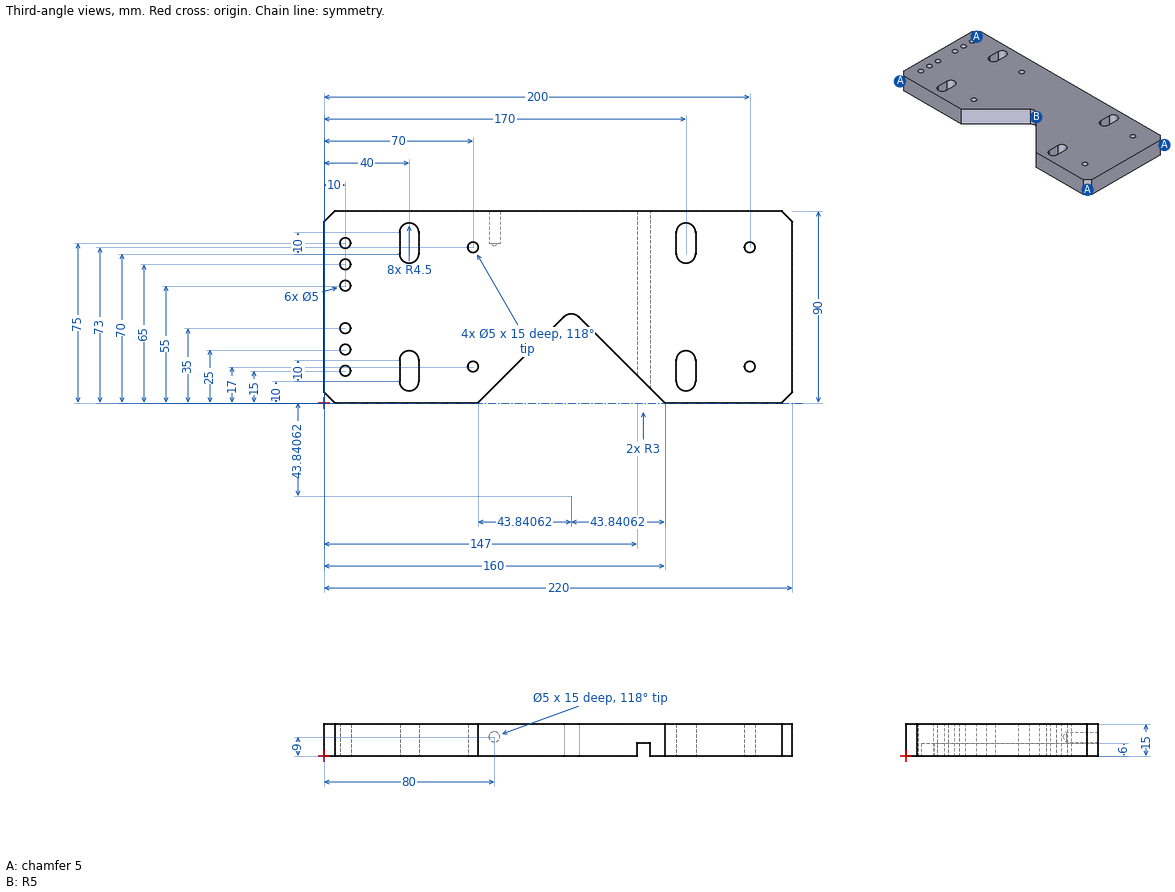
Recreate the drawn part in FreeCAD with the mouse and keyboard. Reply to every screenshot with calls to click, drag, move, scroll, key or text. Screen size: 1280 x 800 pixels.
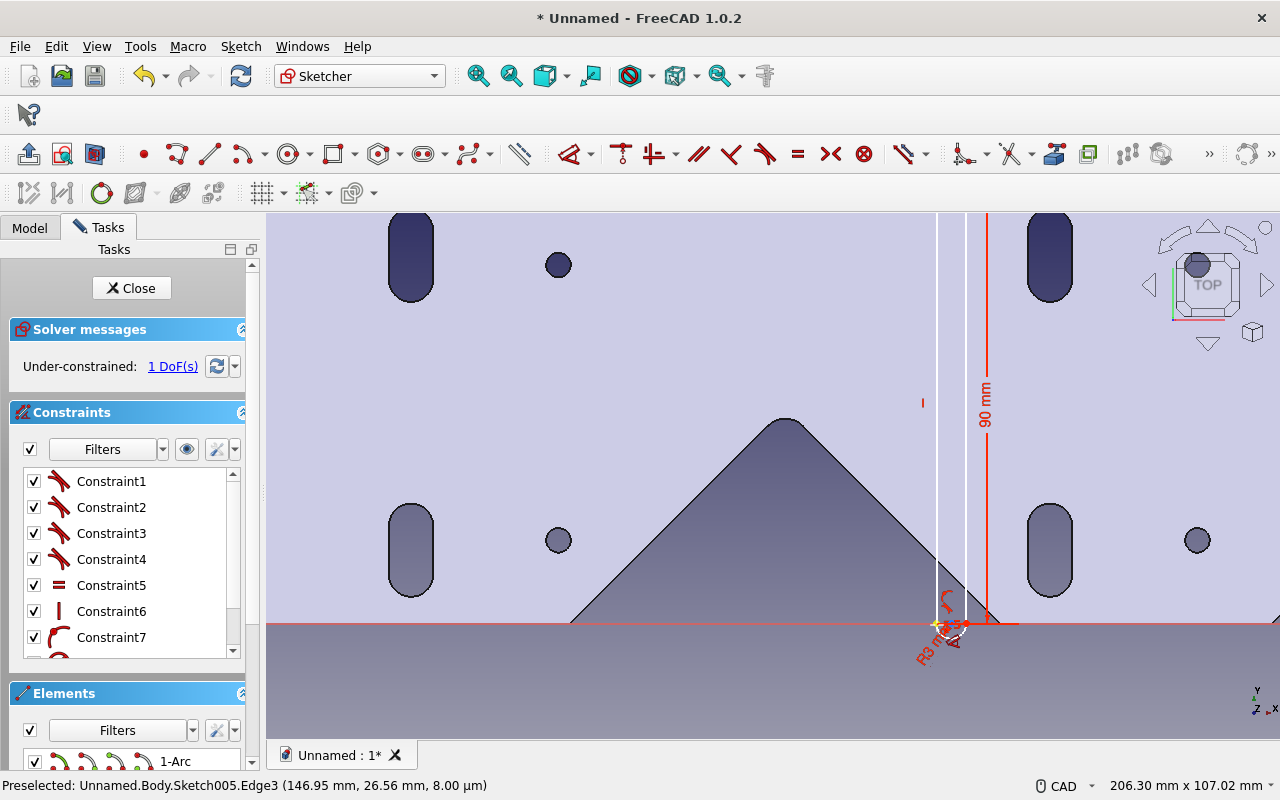
click(937, 624)
click(615, 658)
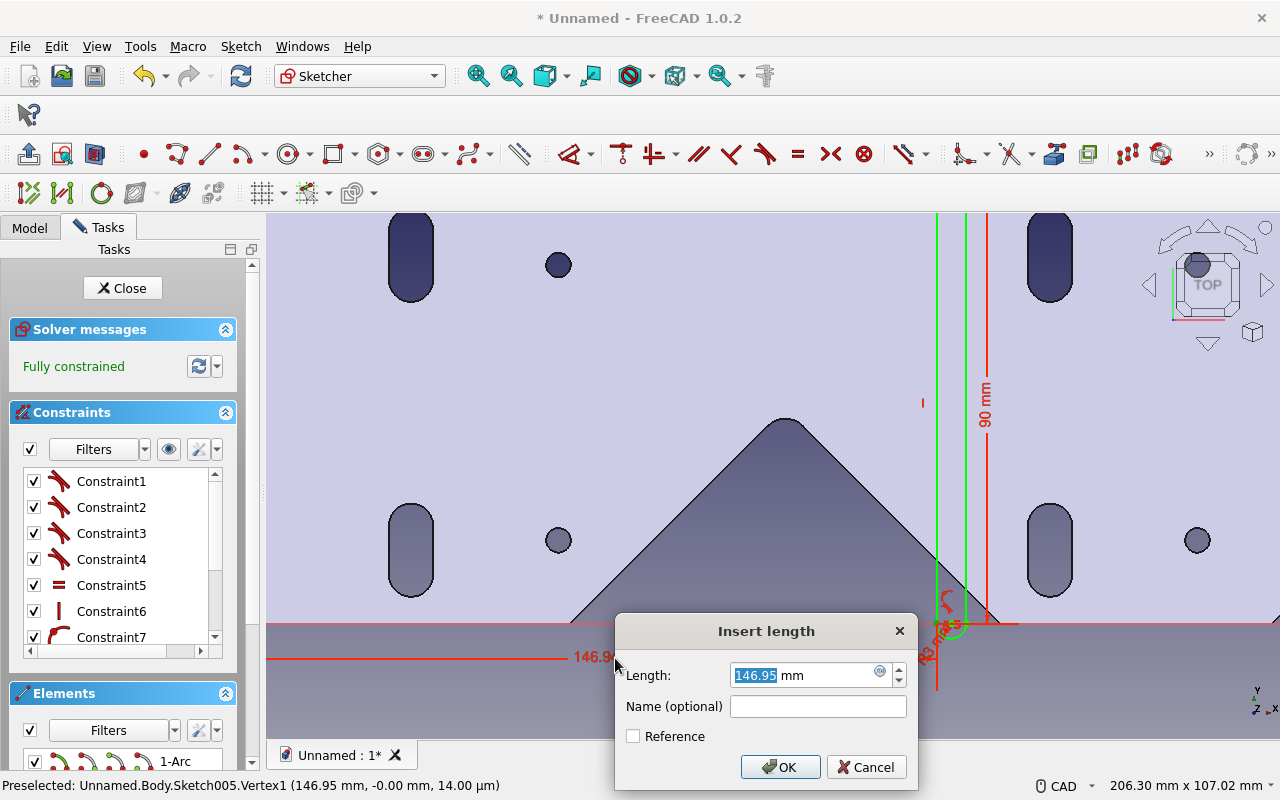
text(147)
key(Return)
key(Escape)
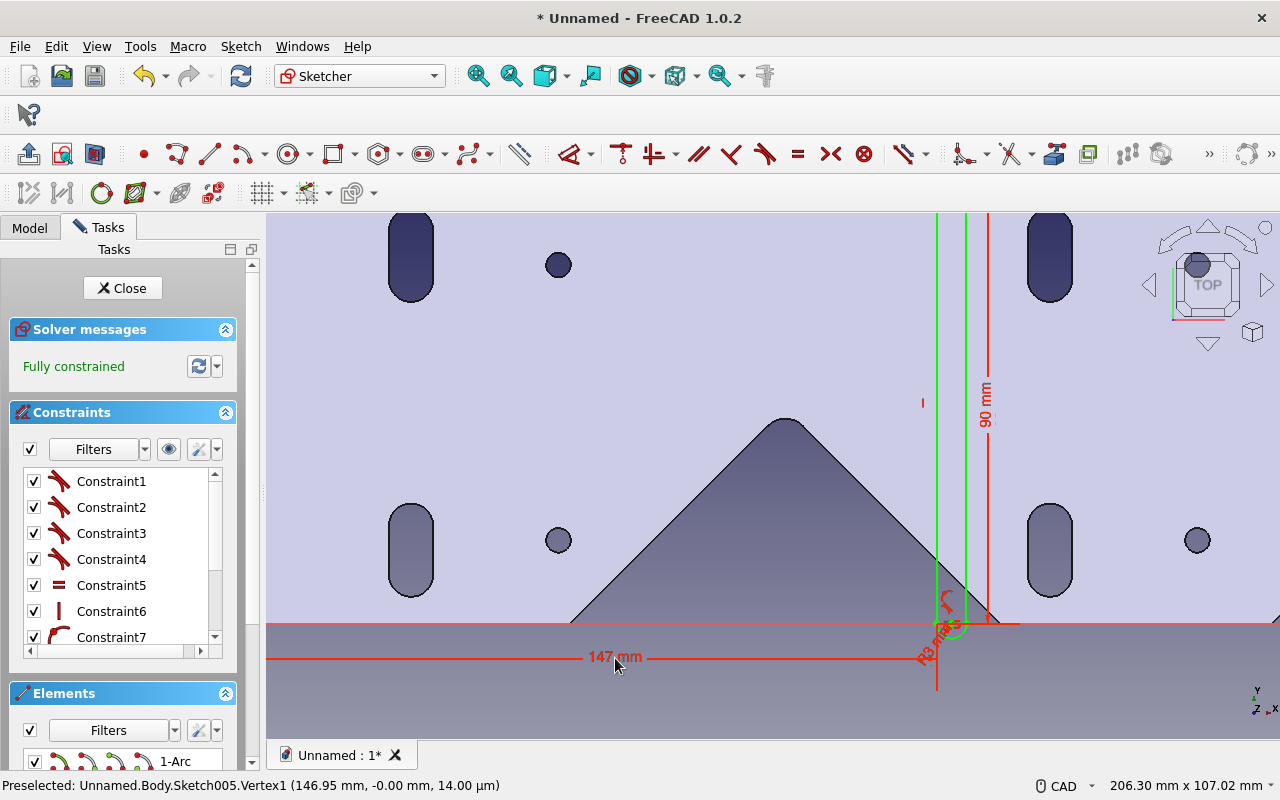
click(123, 288)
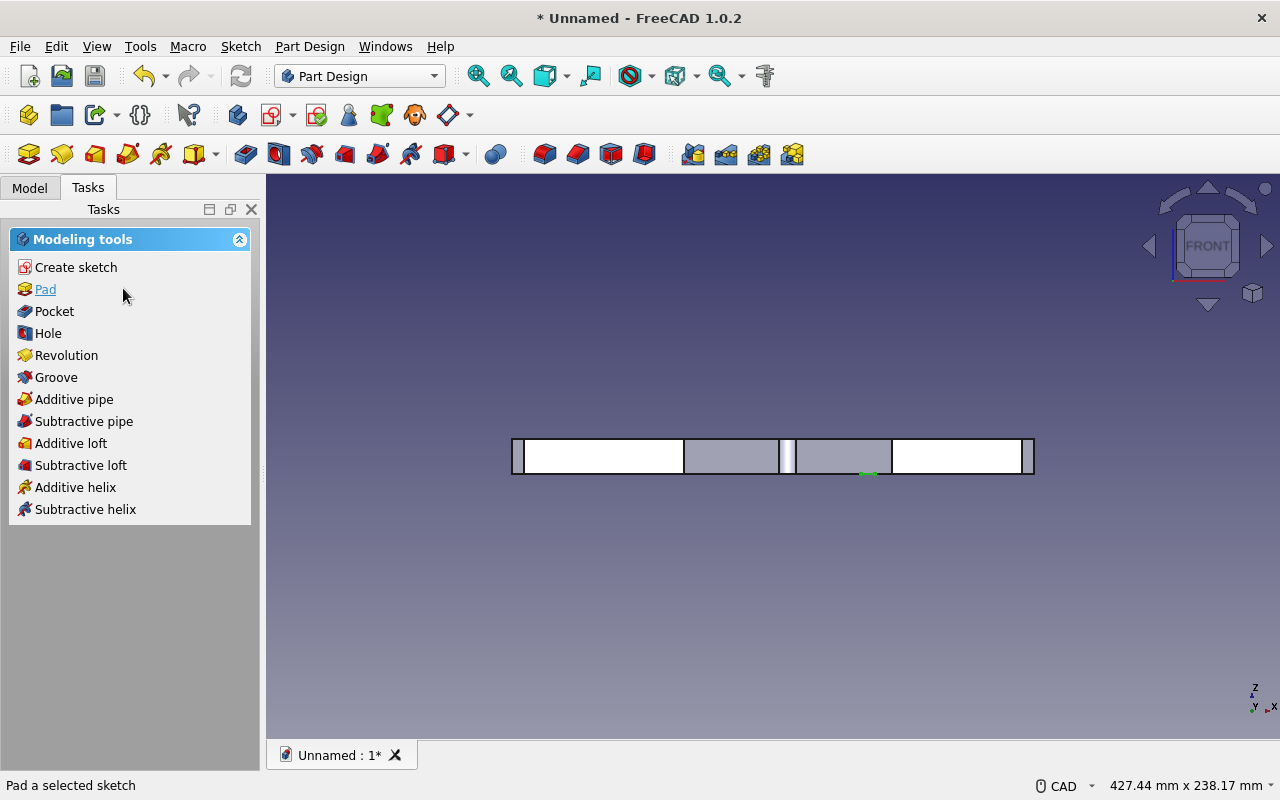
click(246, 154)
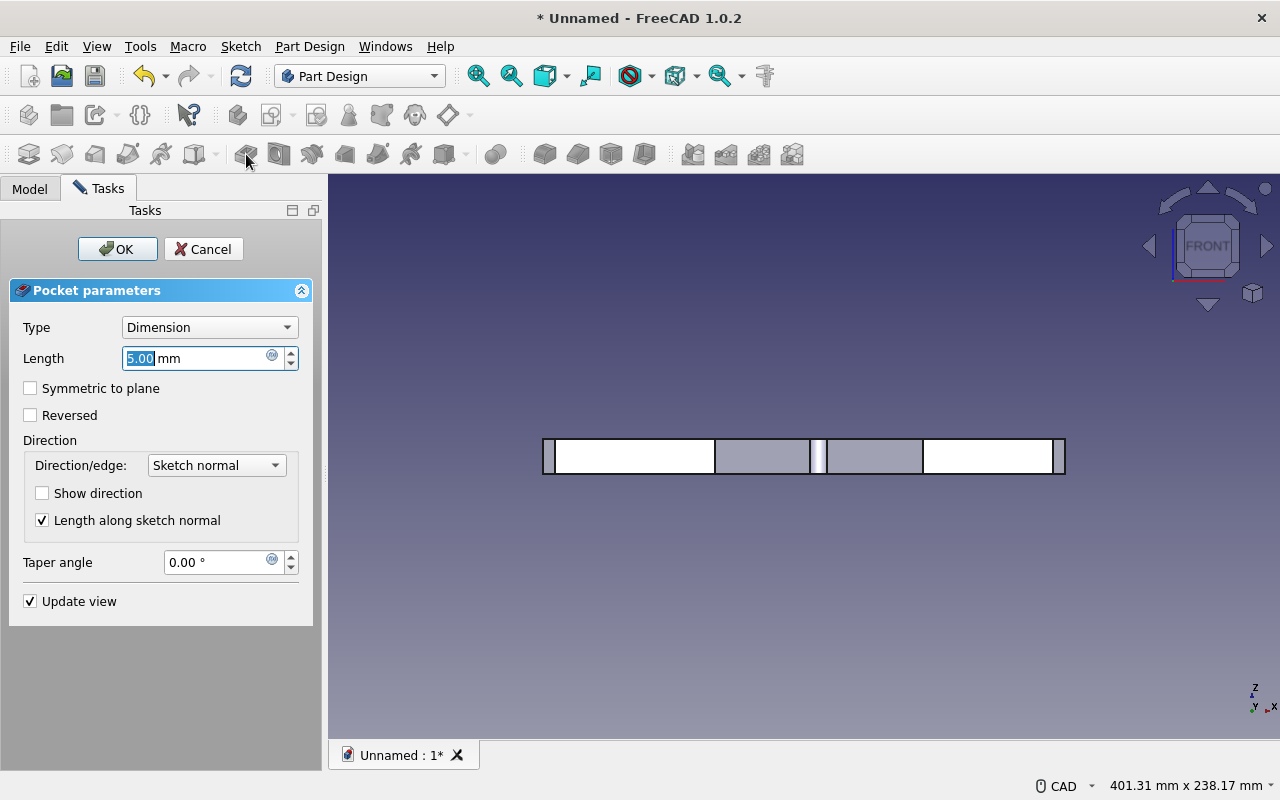
text(6)
key(Tab)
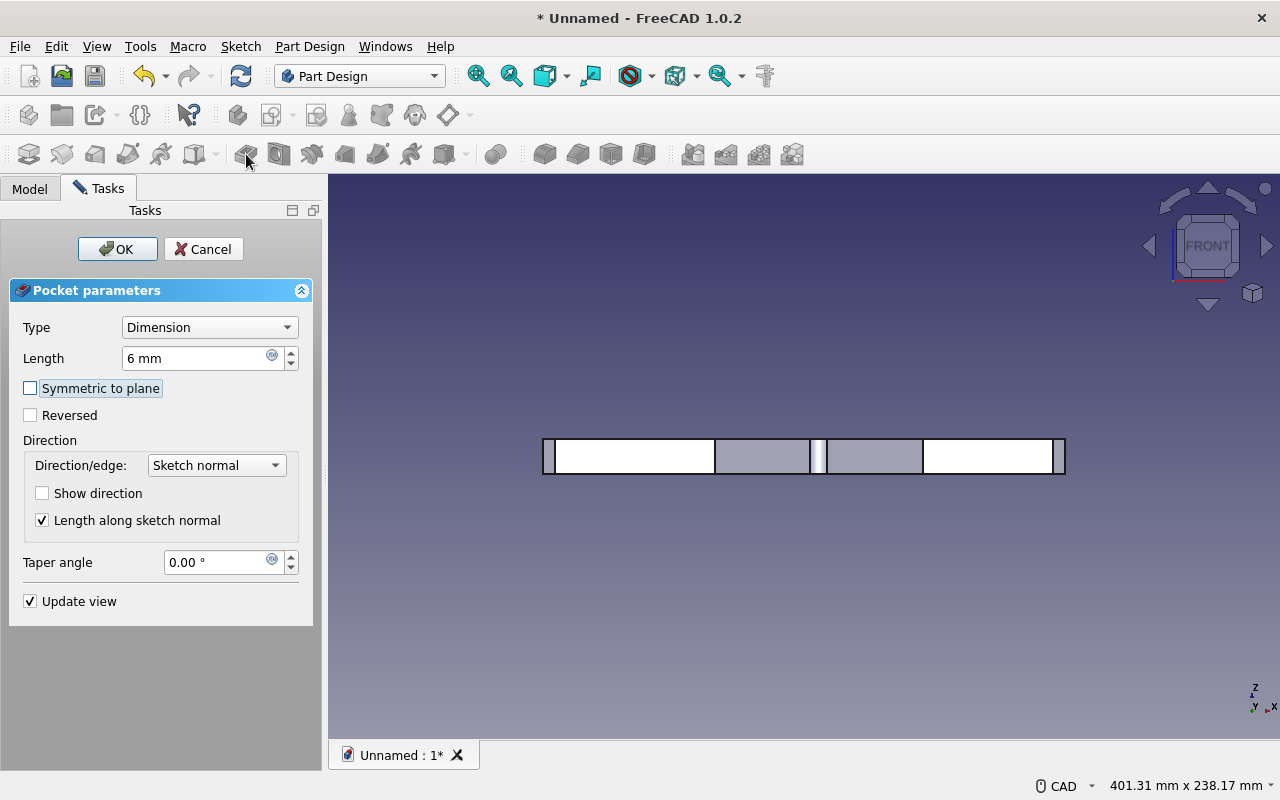
click(31, 415)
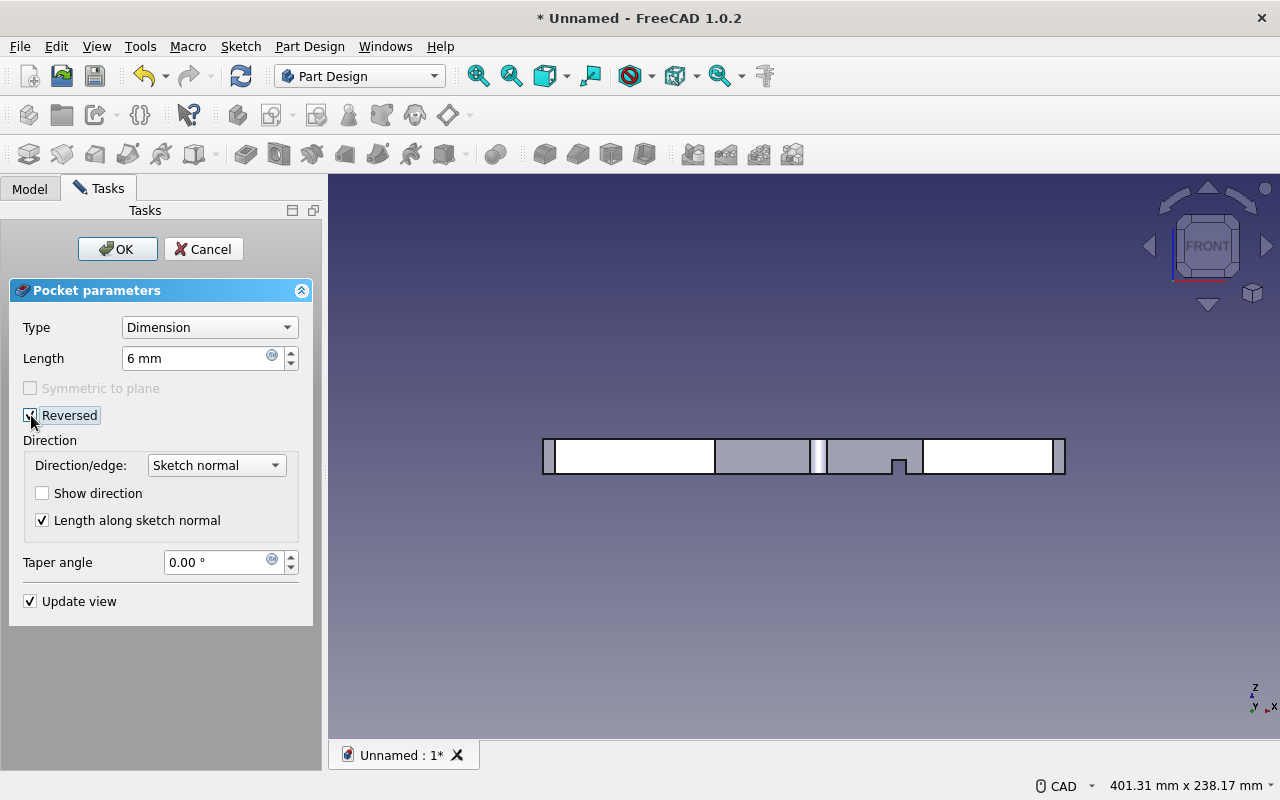
click(118, 249)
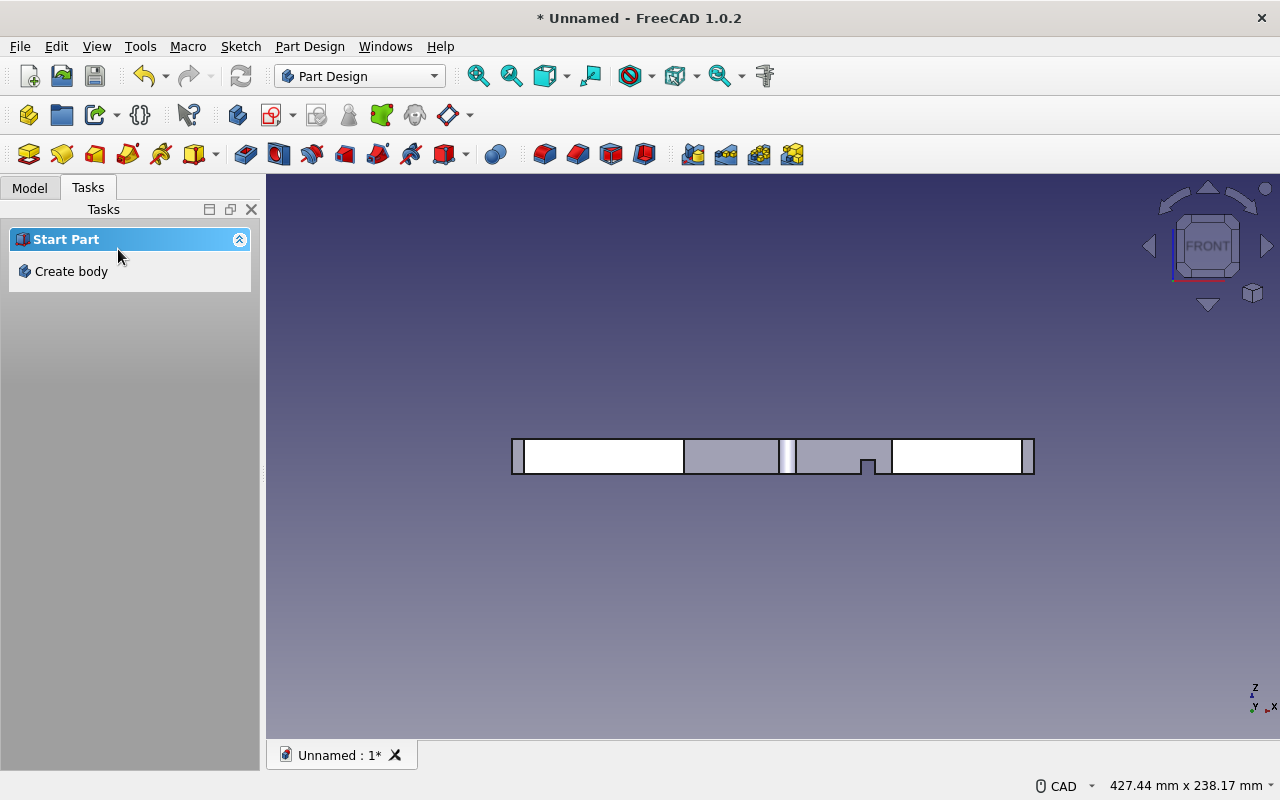
key(0)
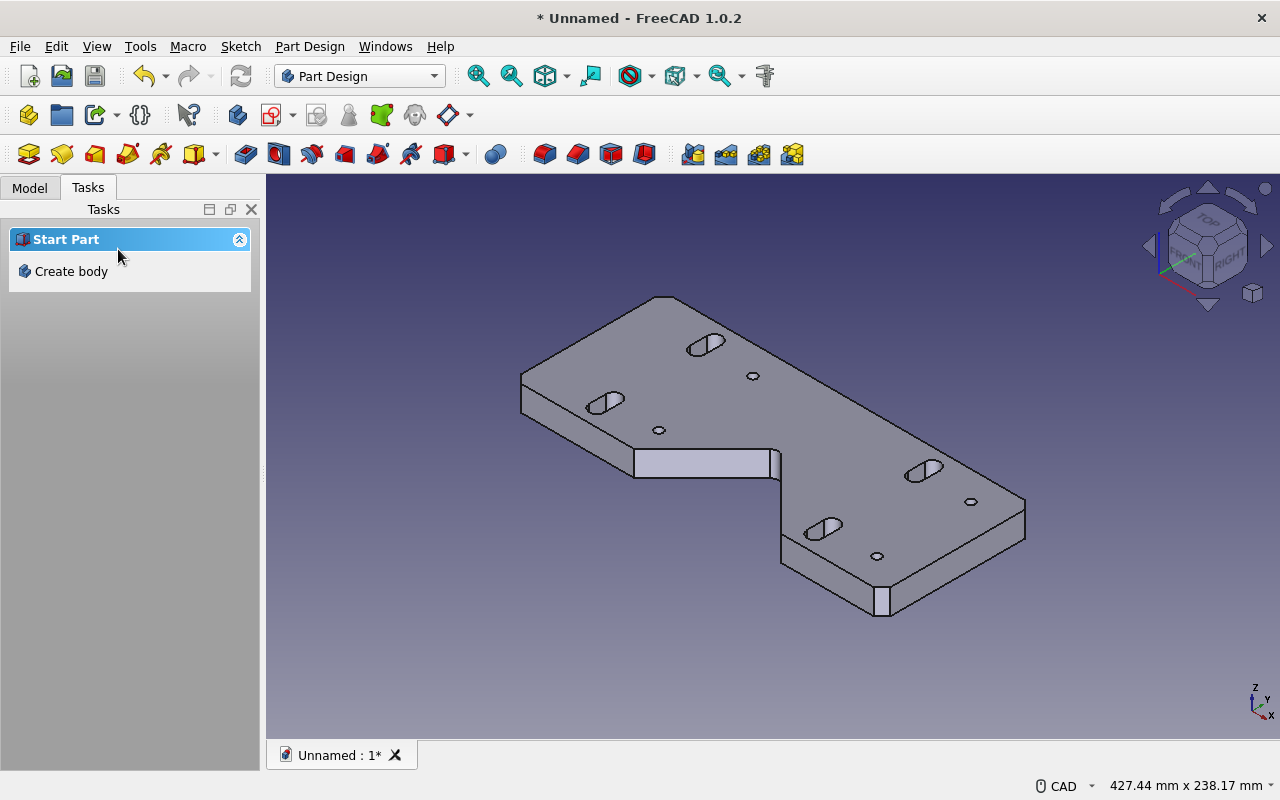
click(720, 411)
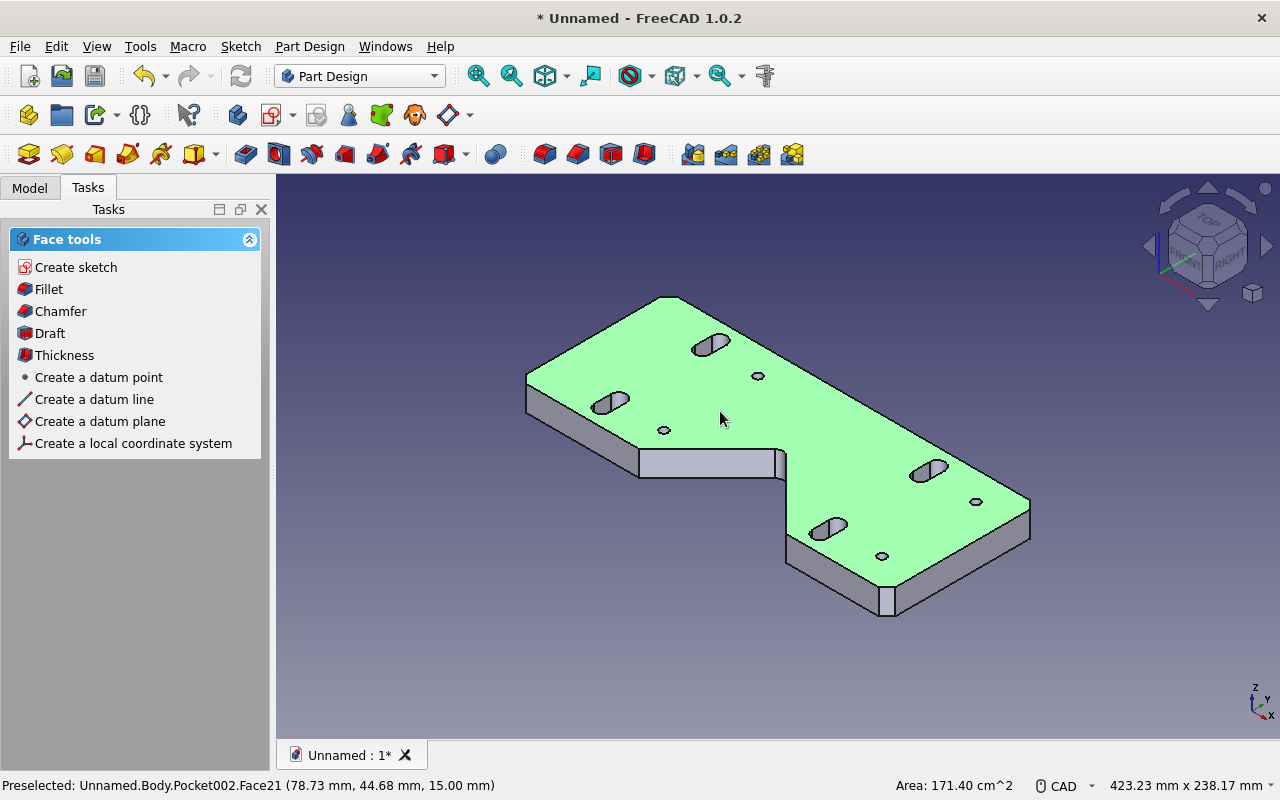
click(270, 116)